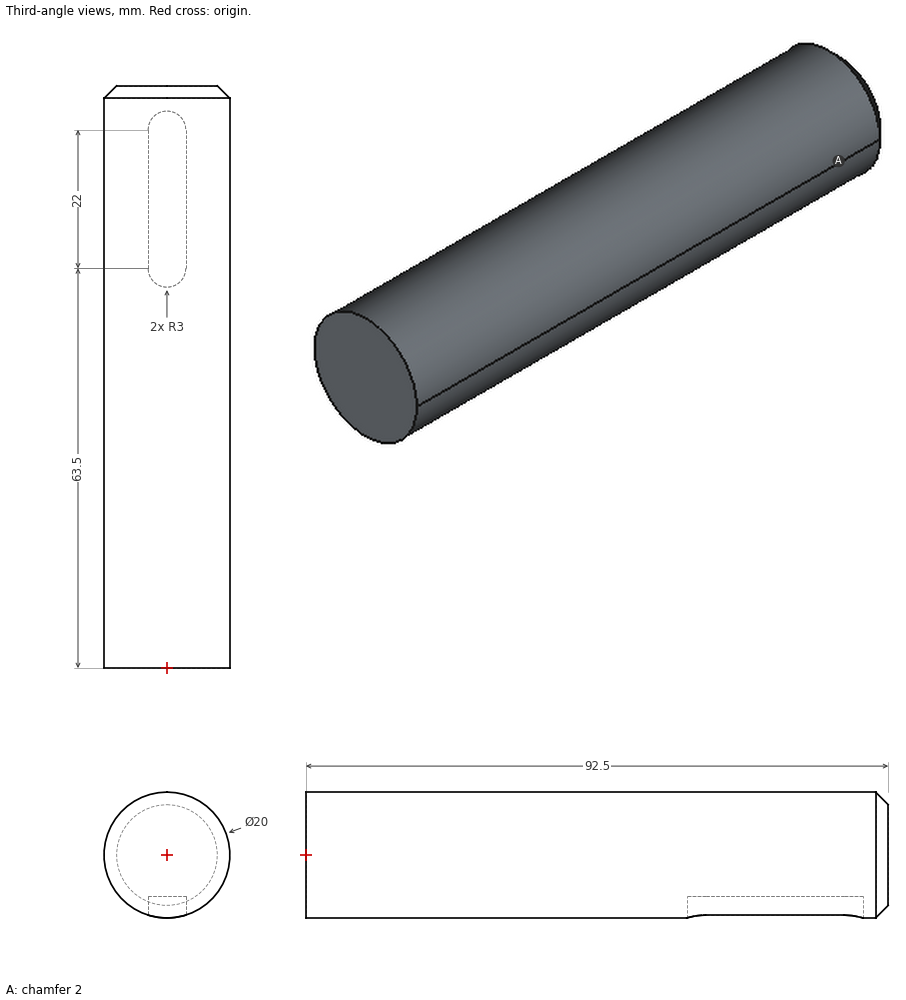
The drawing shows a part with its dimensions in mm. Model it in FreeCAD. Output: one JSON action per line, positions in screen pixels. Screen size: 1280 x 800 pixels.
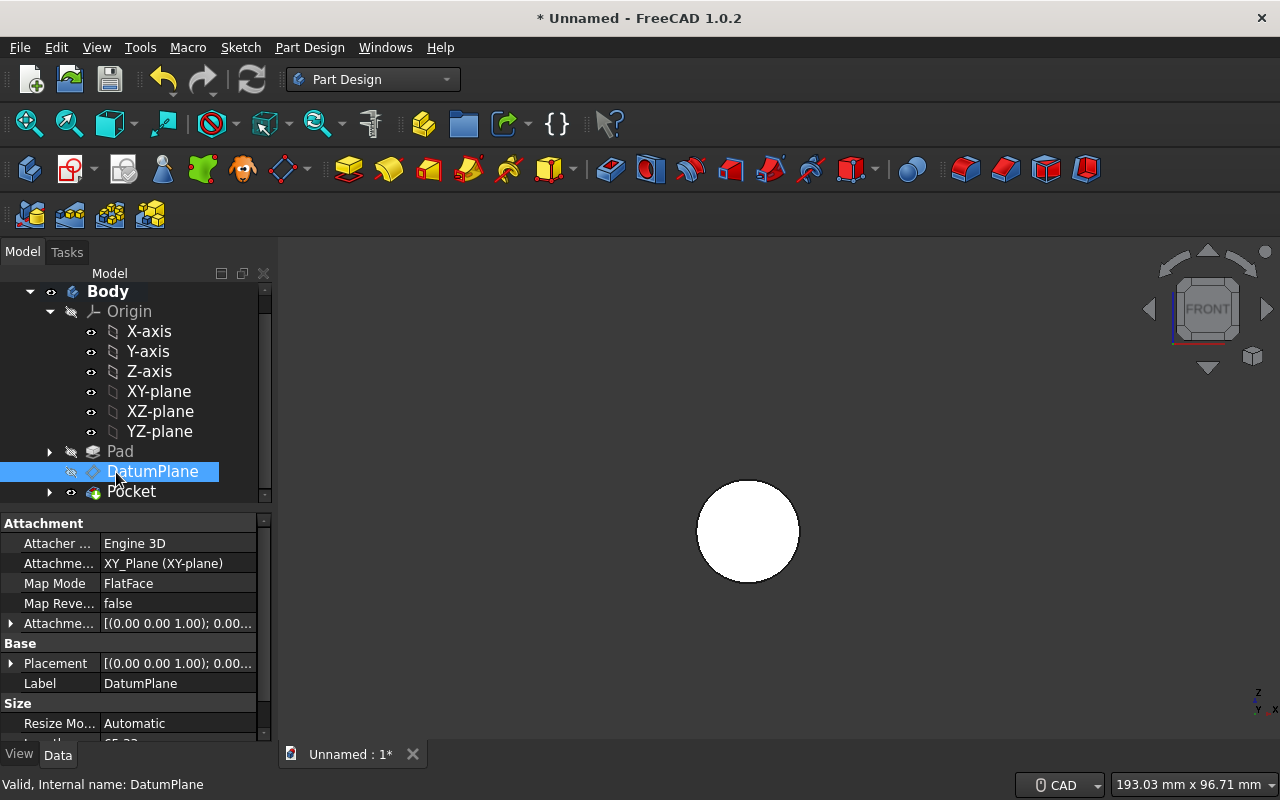
{"action": "key", "text": "v f"}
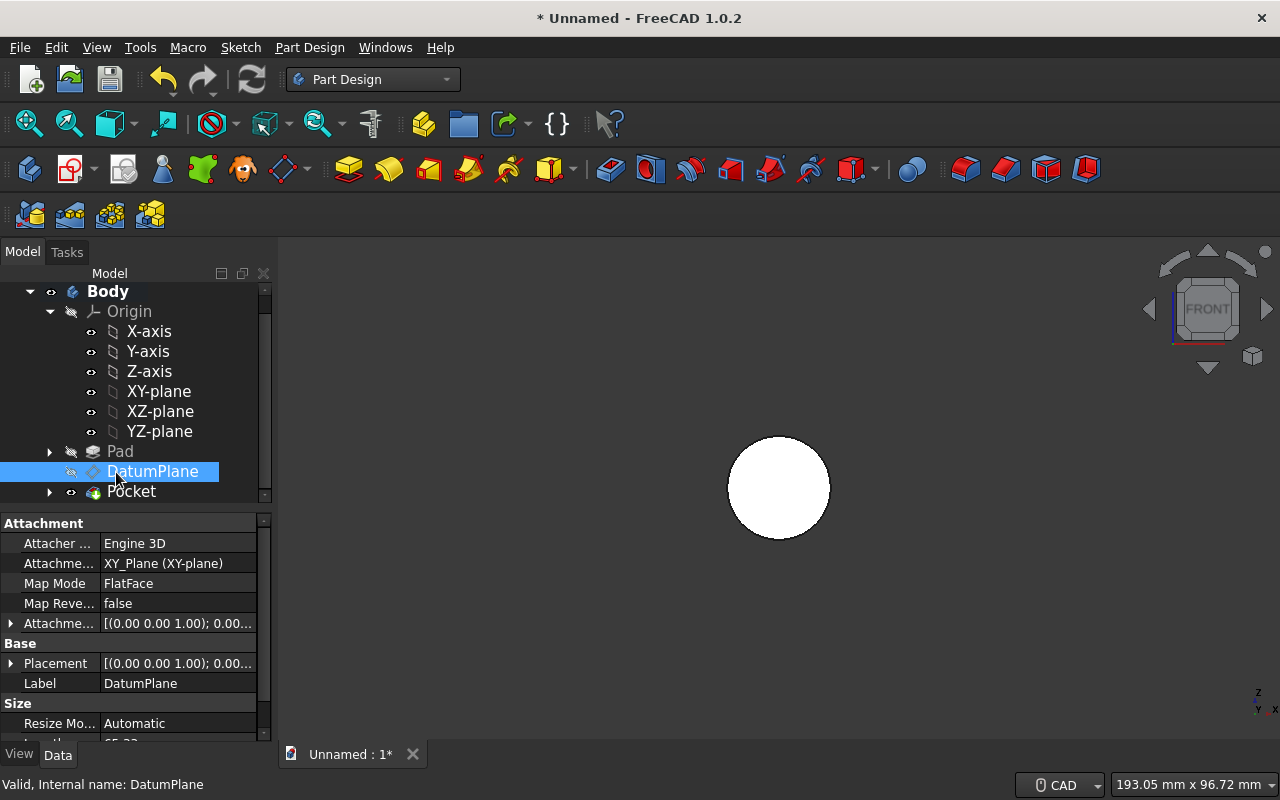
{"action": "key", "text": "3"}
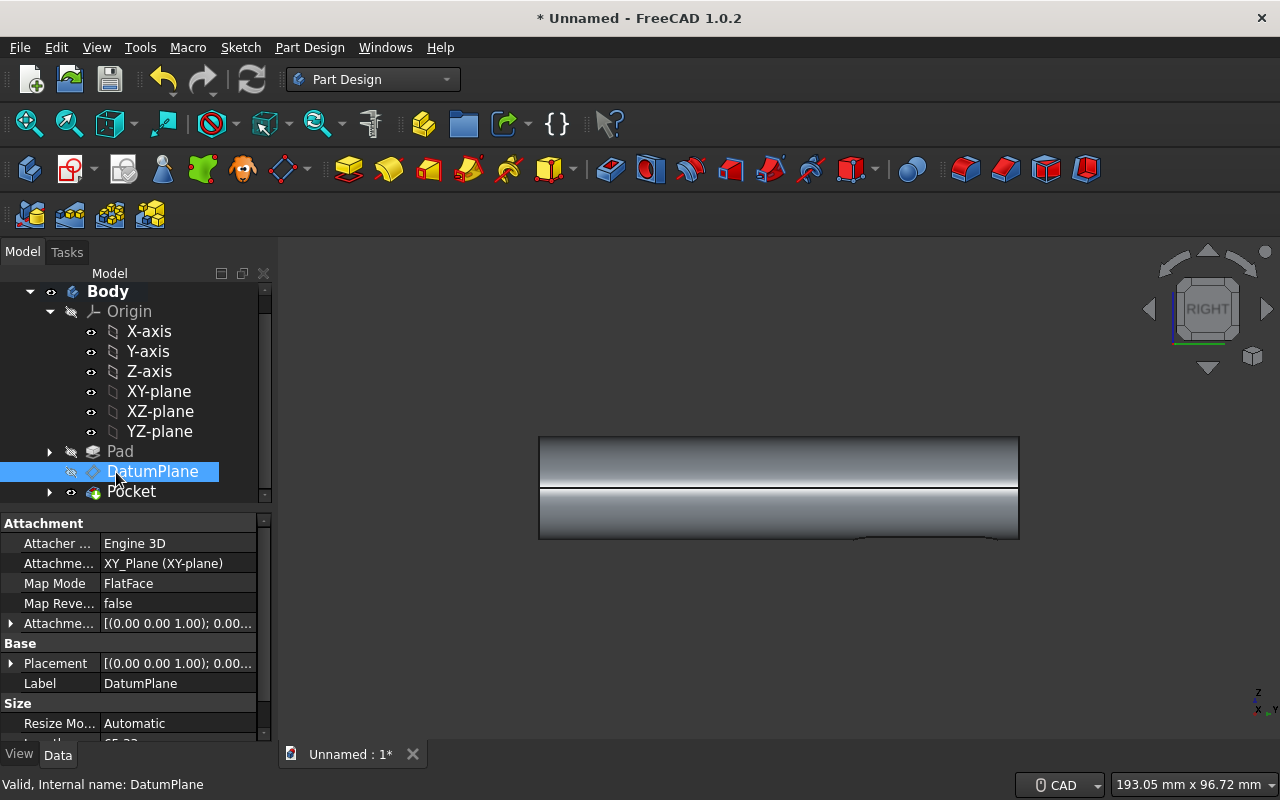
{"action": "left_click", "coordinate": [1019, 456]}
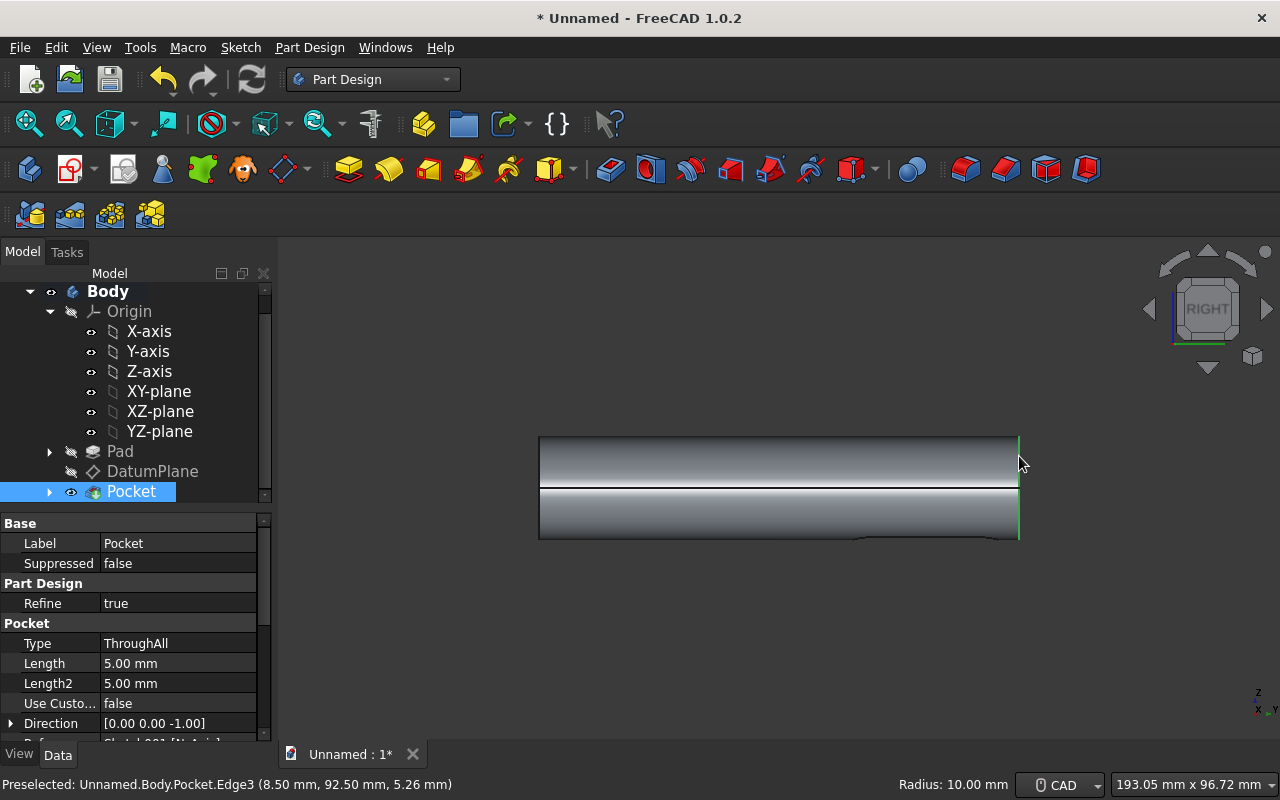
{"action": "left_click", "coordinate": [1006, 170]}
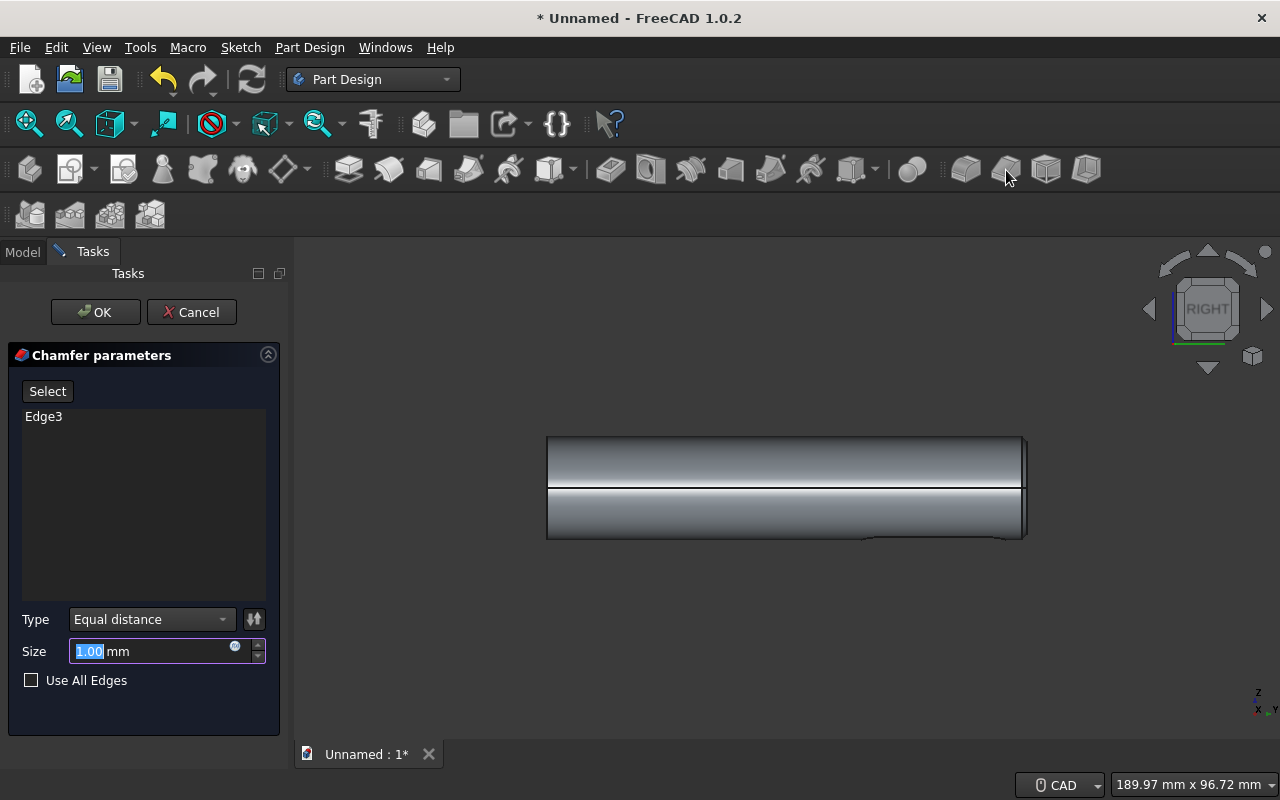
{"action": "type", "text": "2"}
{"action": "key", "text": "Tab"}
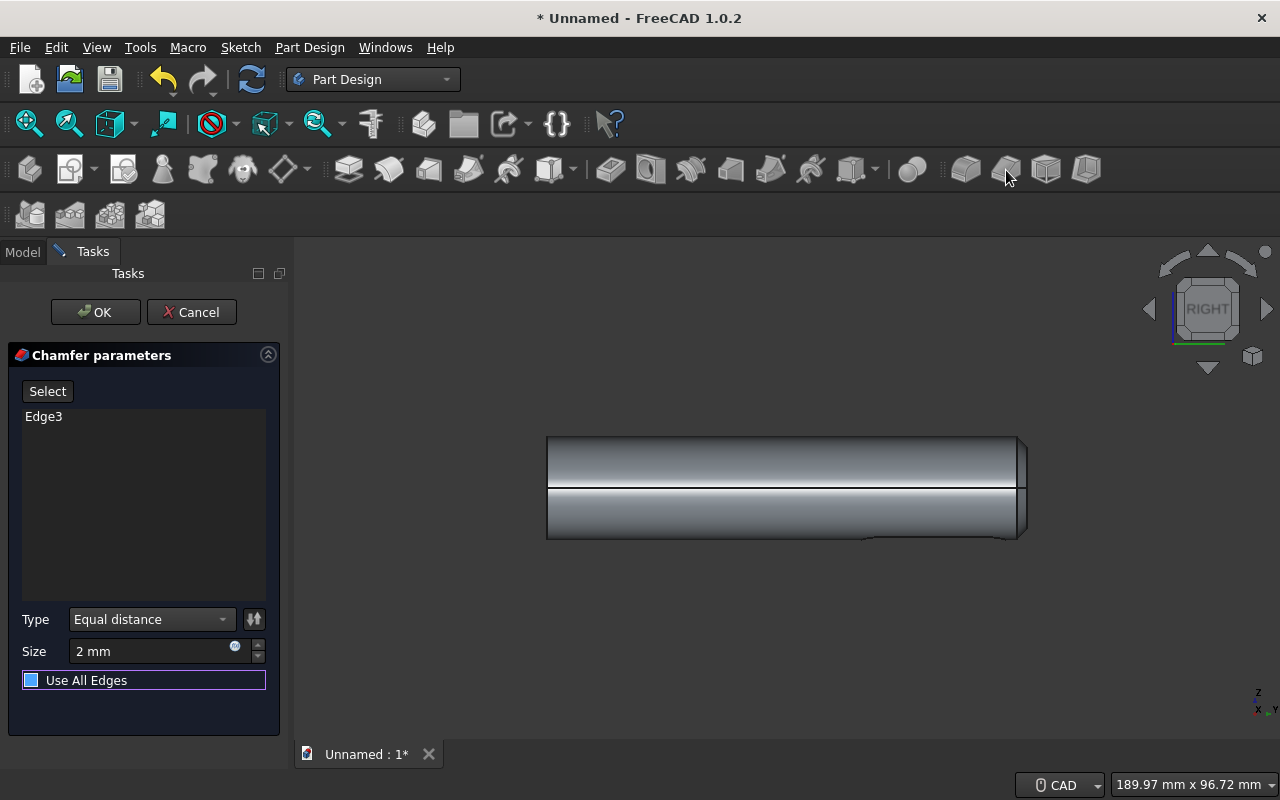
{"action": "left_click", "coordinate": [96, 312]}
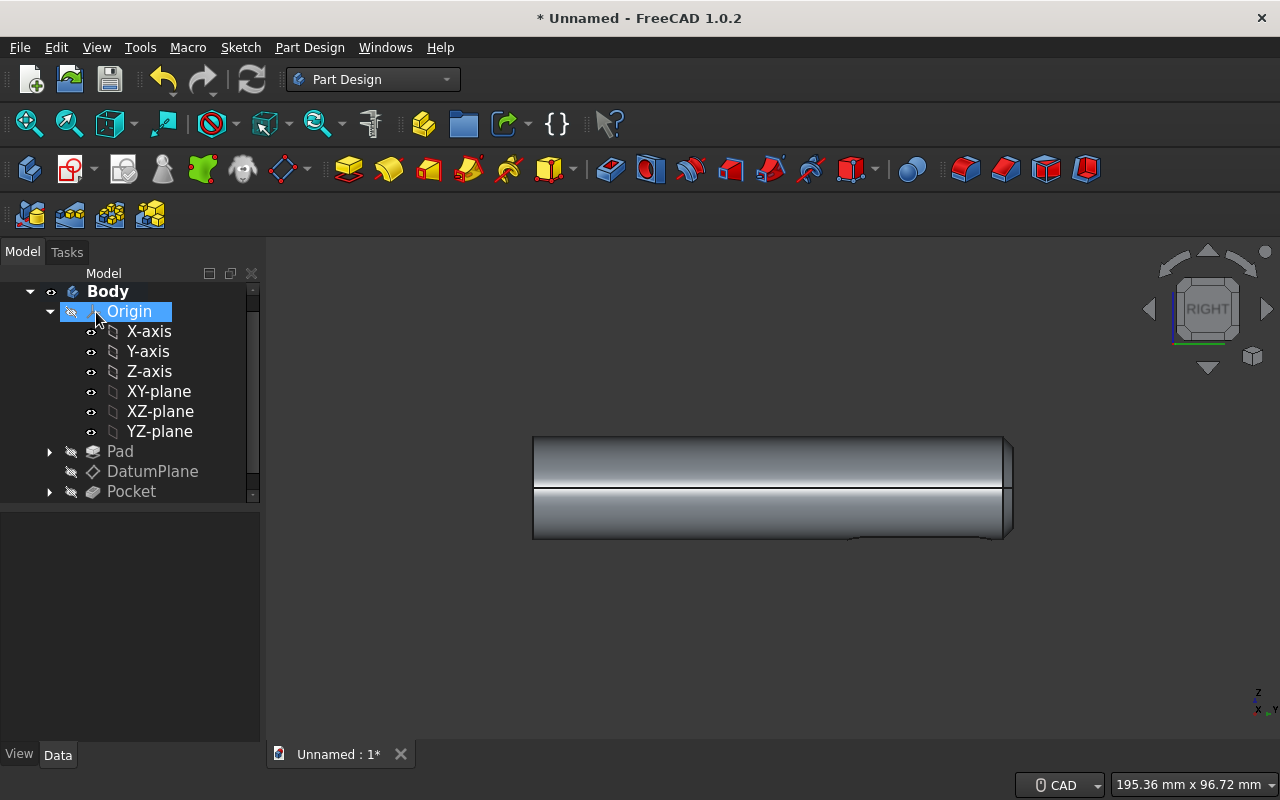
{"action": "key", "text": "0"}